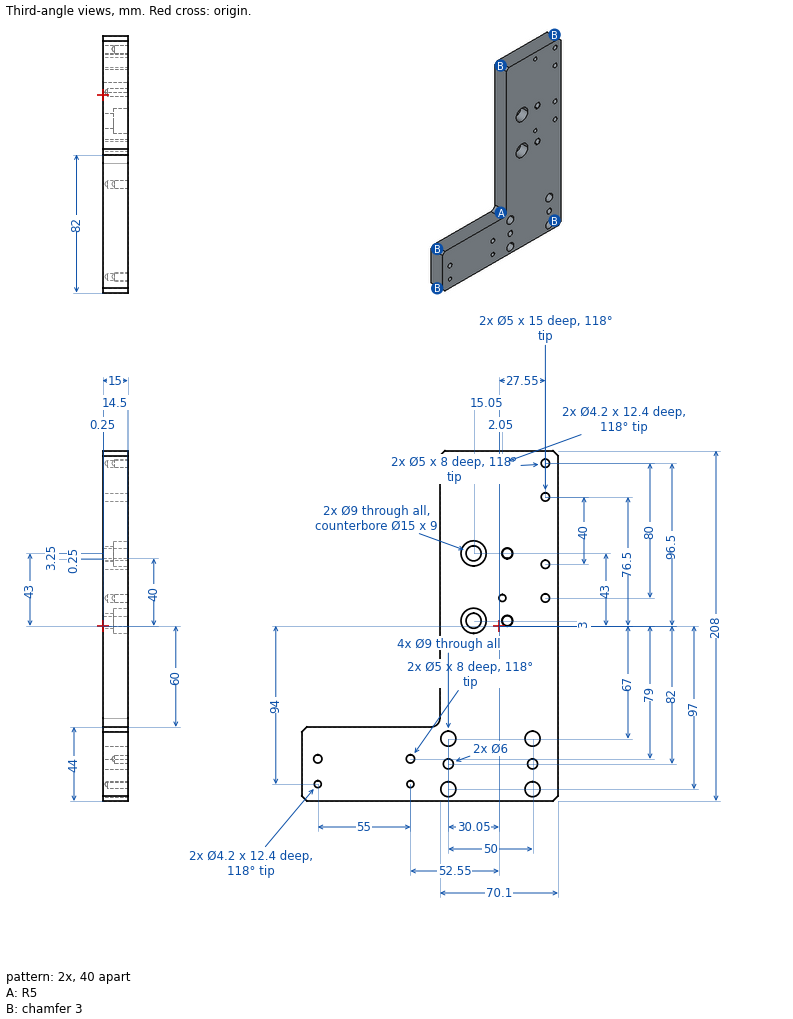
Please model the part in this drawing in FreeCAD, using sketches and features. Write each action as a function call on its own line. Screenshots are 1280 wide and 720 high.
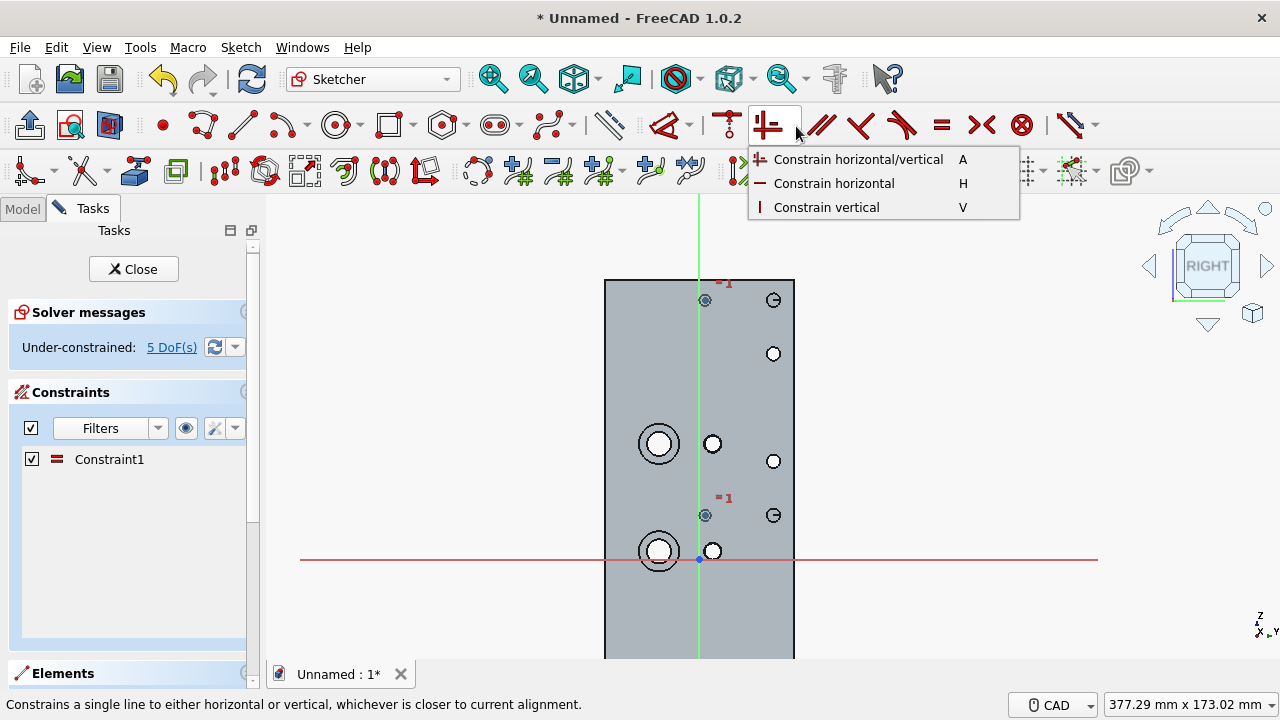
click(884, 207)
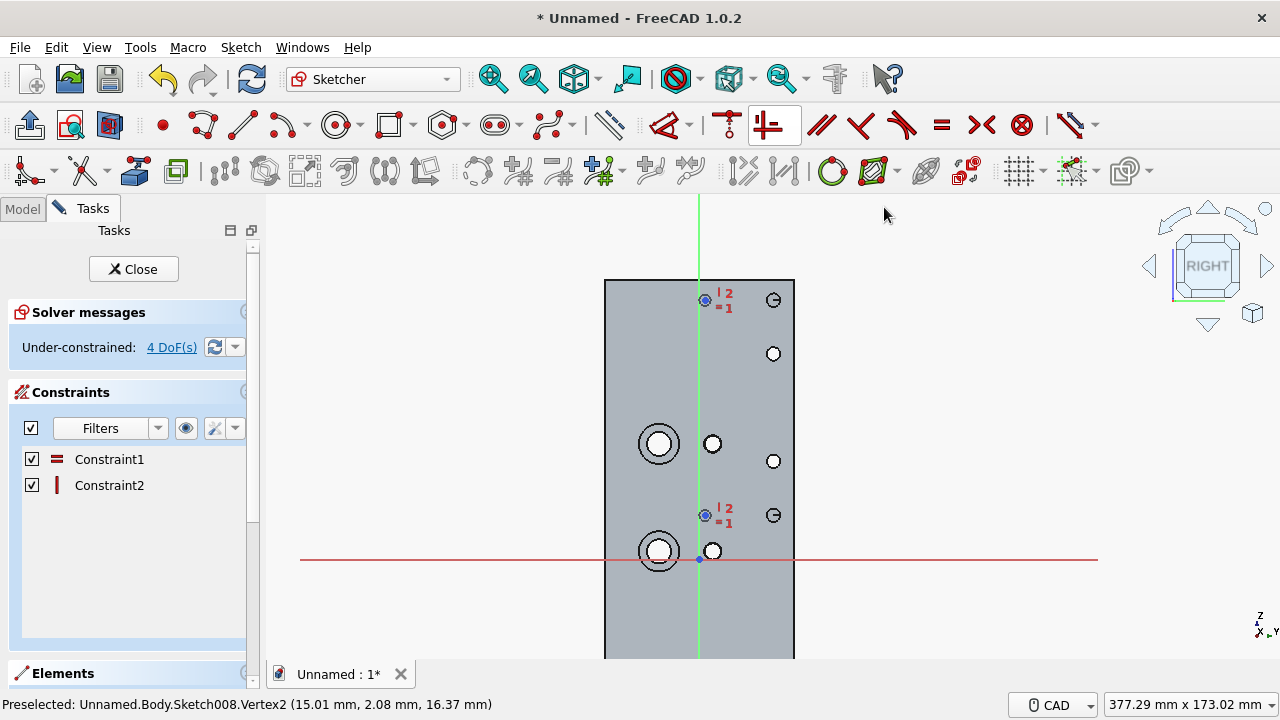
click(664, 126)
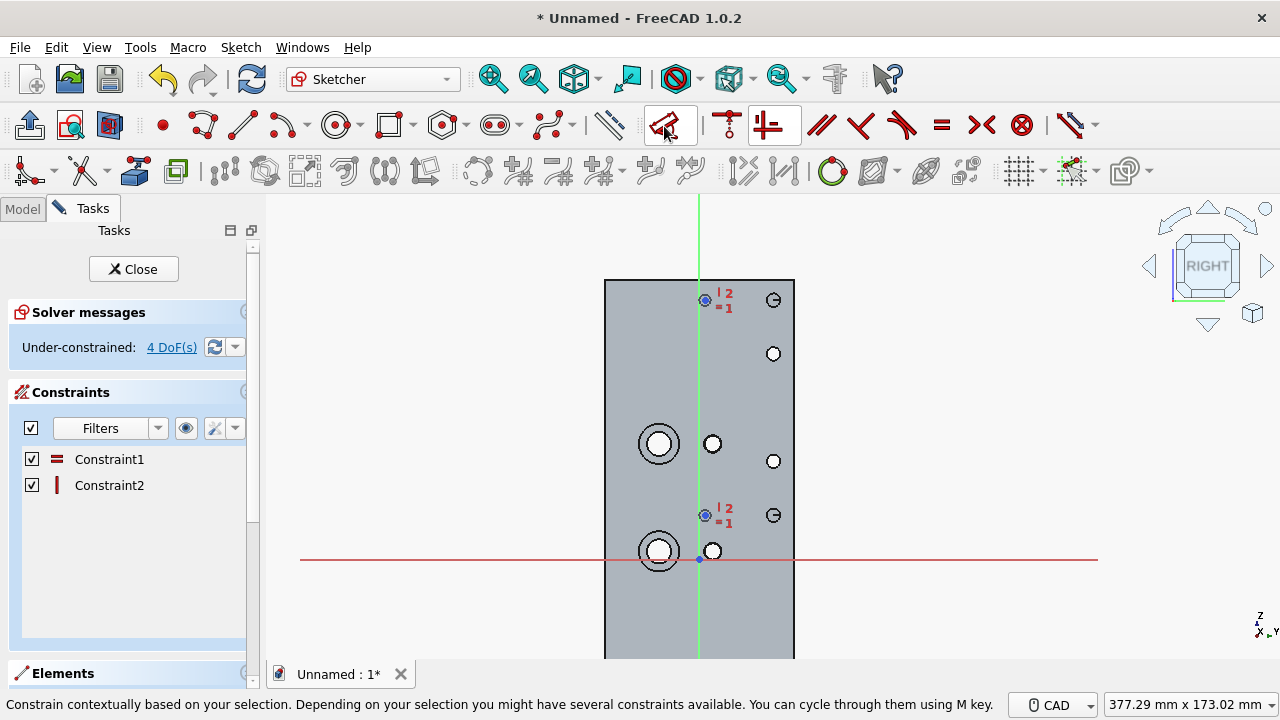
scroll(701, 304, up, 7)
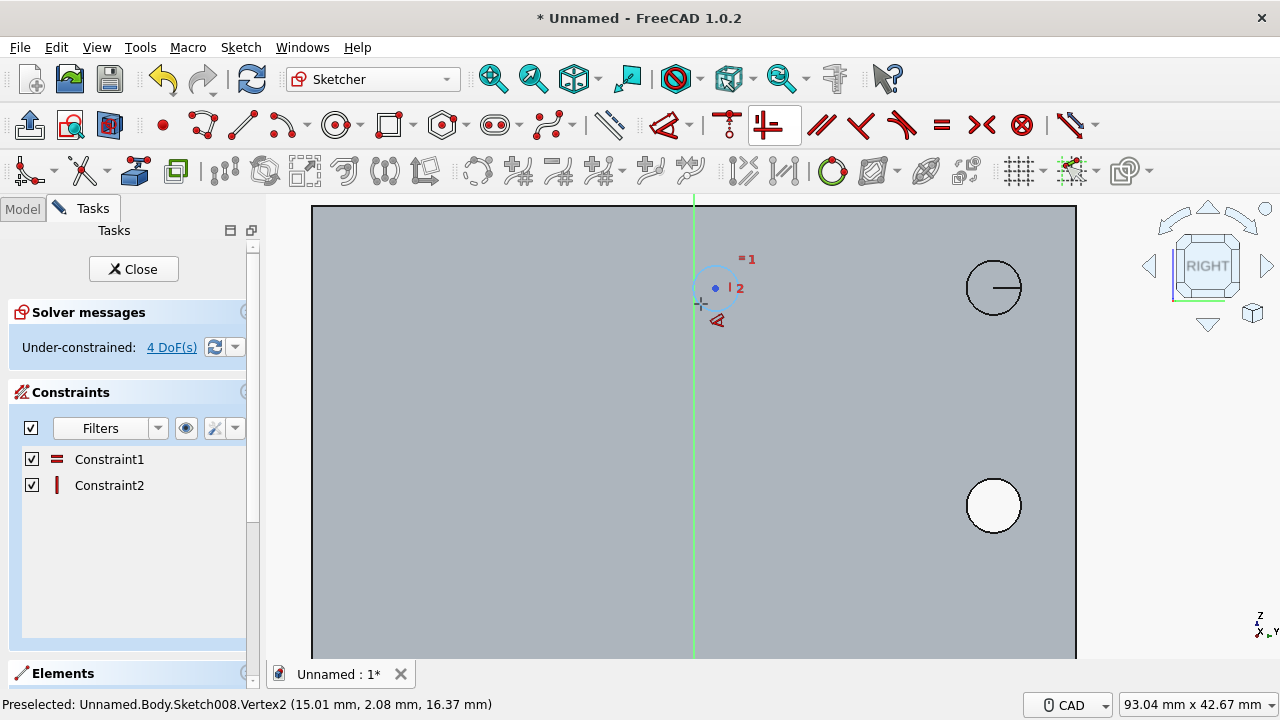
click(700, 304)
click(677, 326)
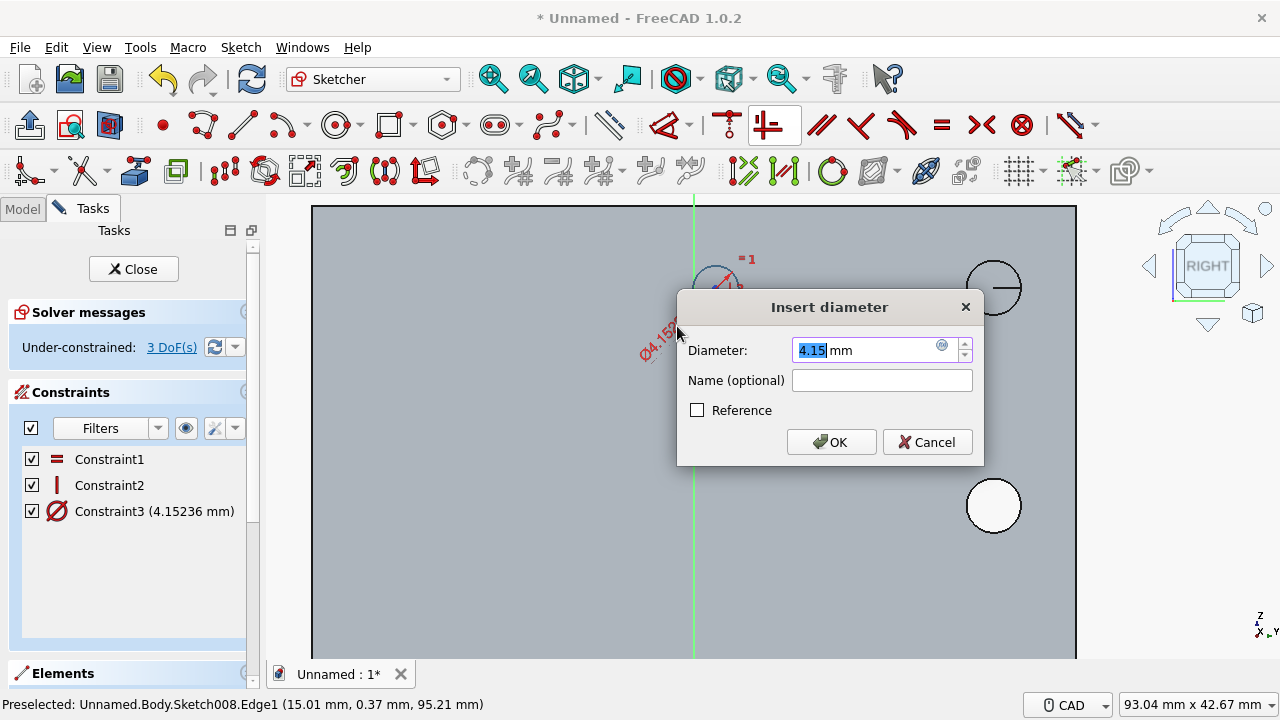
text(4.2)
key(Return)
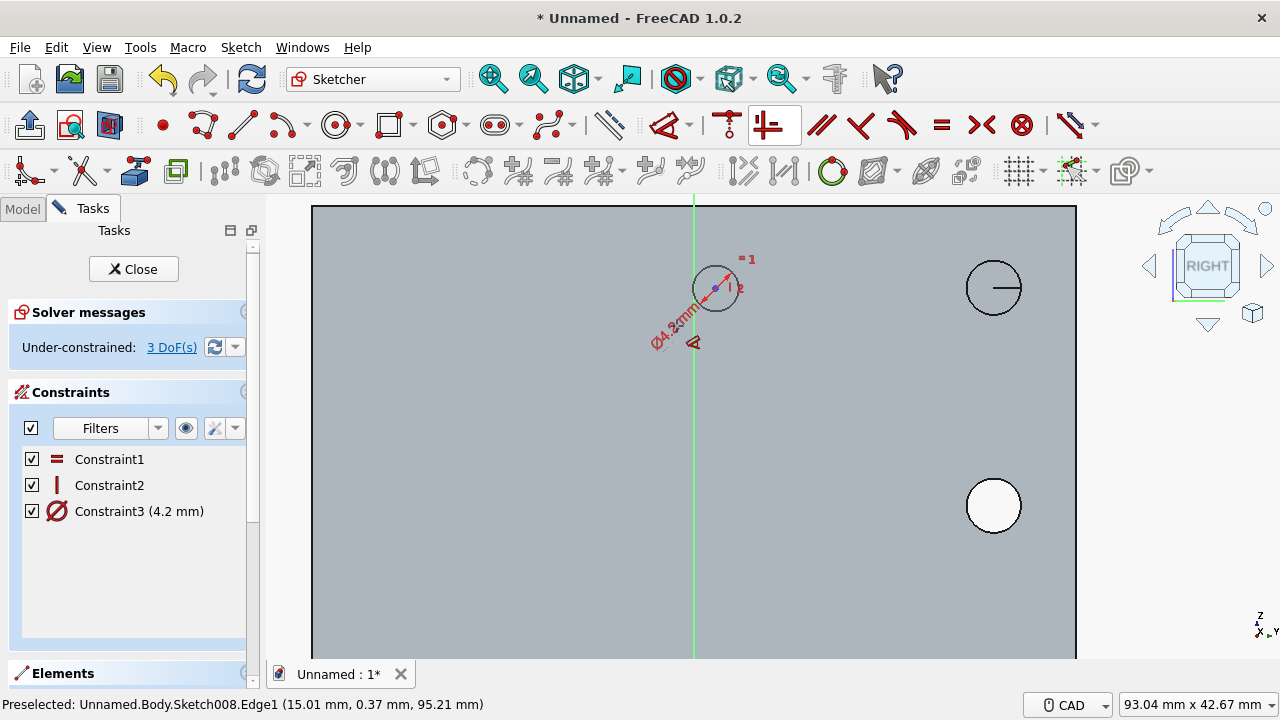
scroll(701, 304, down, 7)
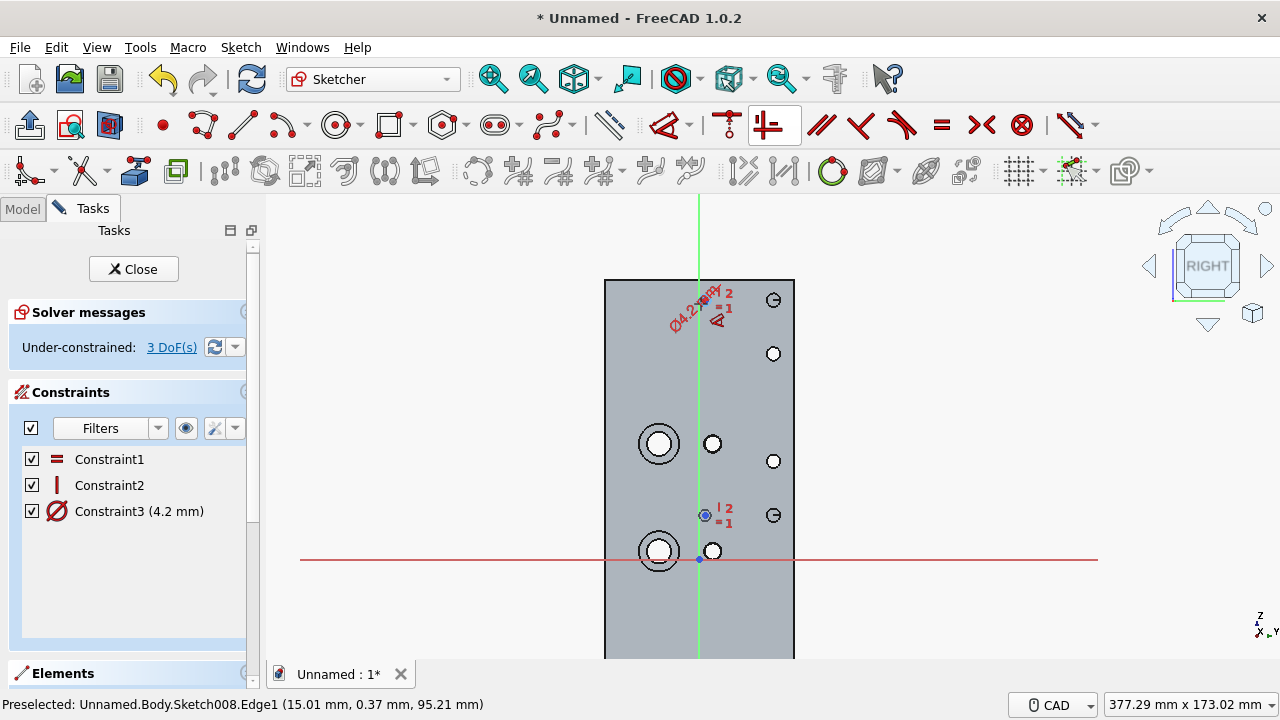
click(705, 300)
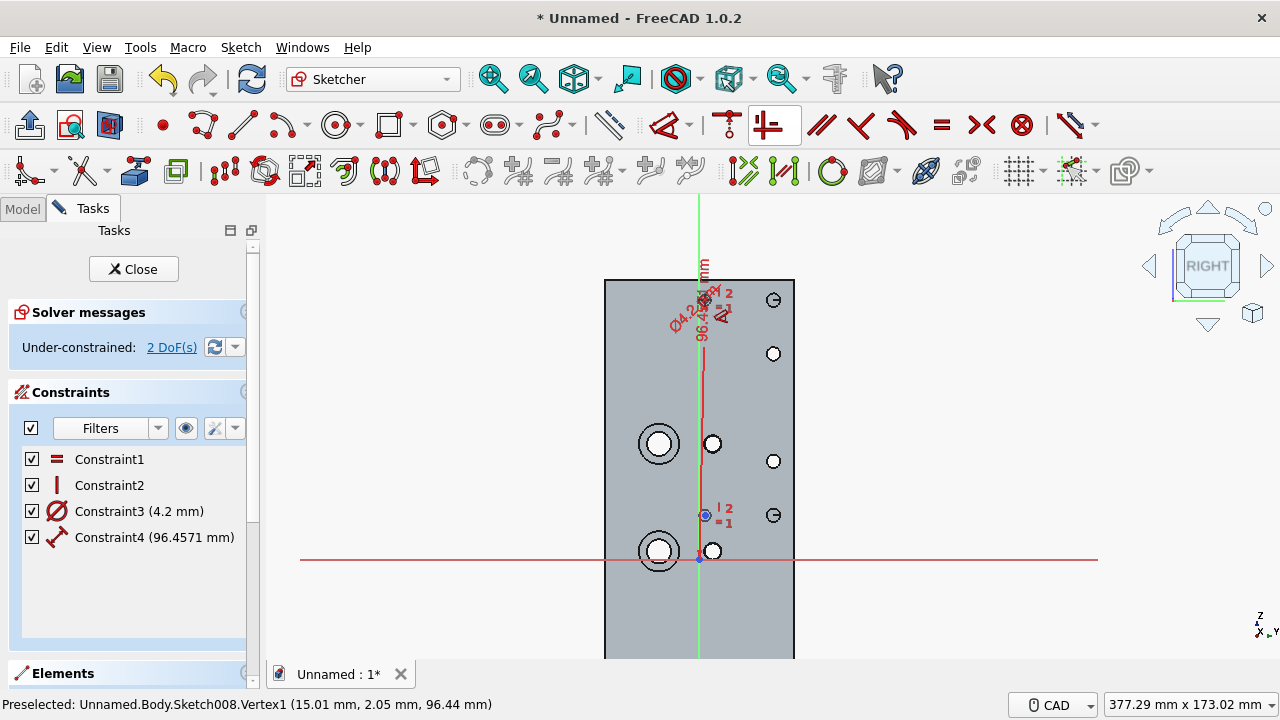
click(705, 516)
click(739, 408)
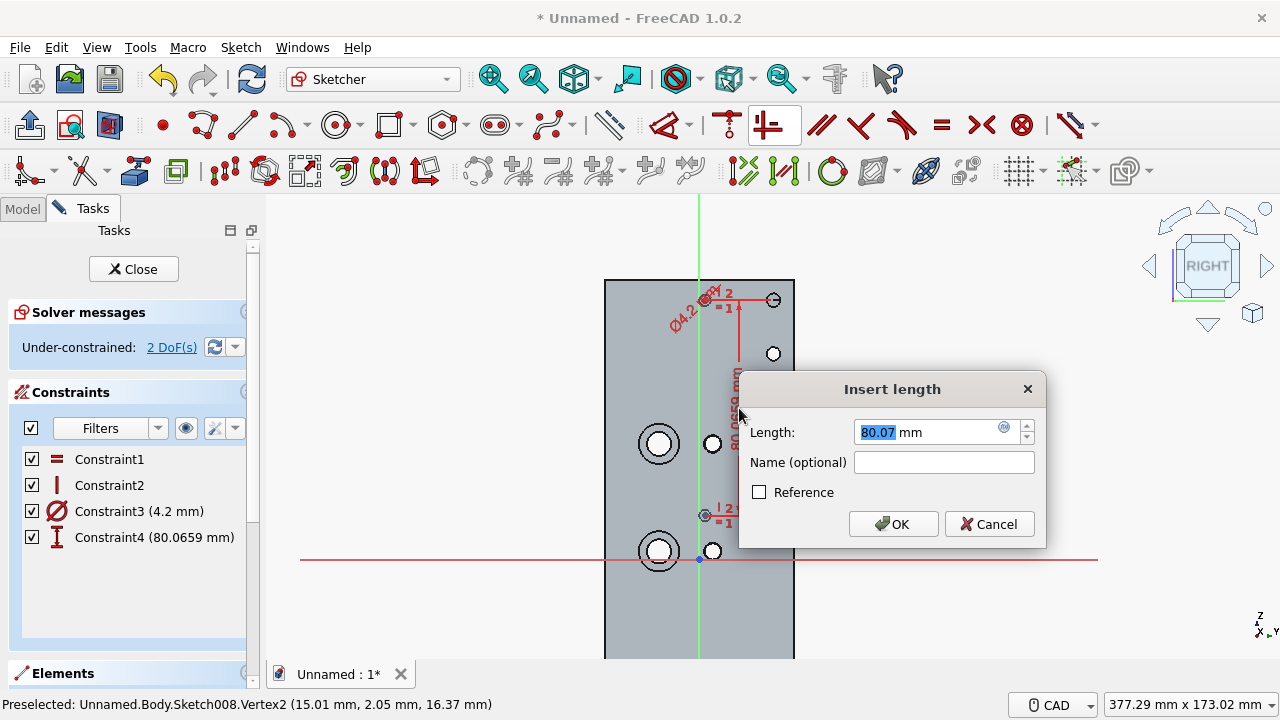
text(80)
key(Return)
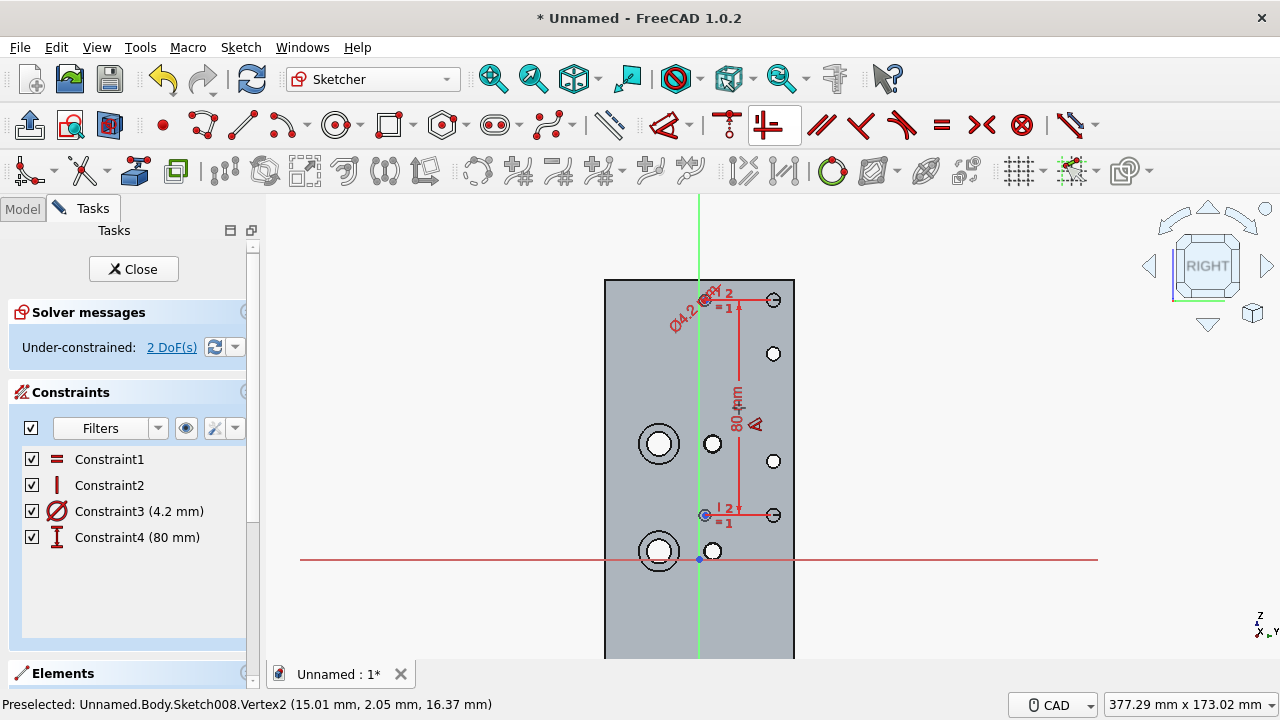
scroll(705, 300, up, 10)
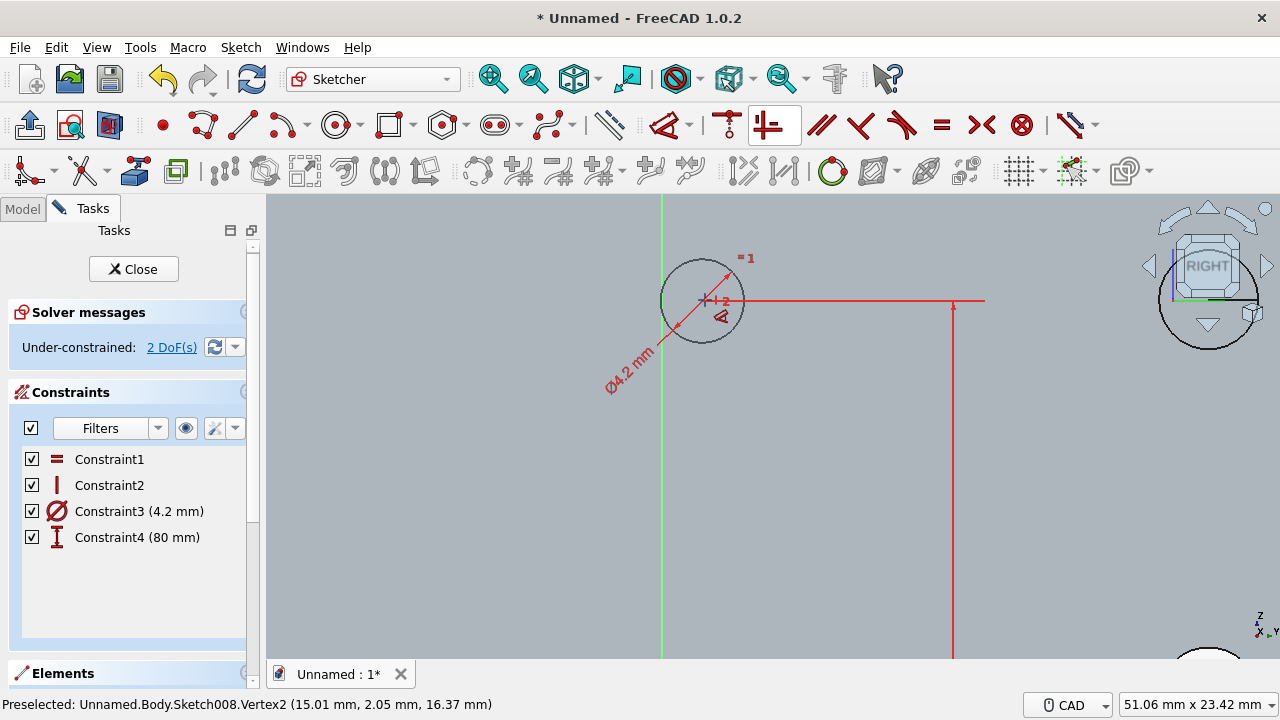
click(702, 301)
click(682, 243)